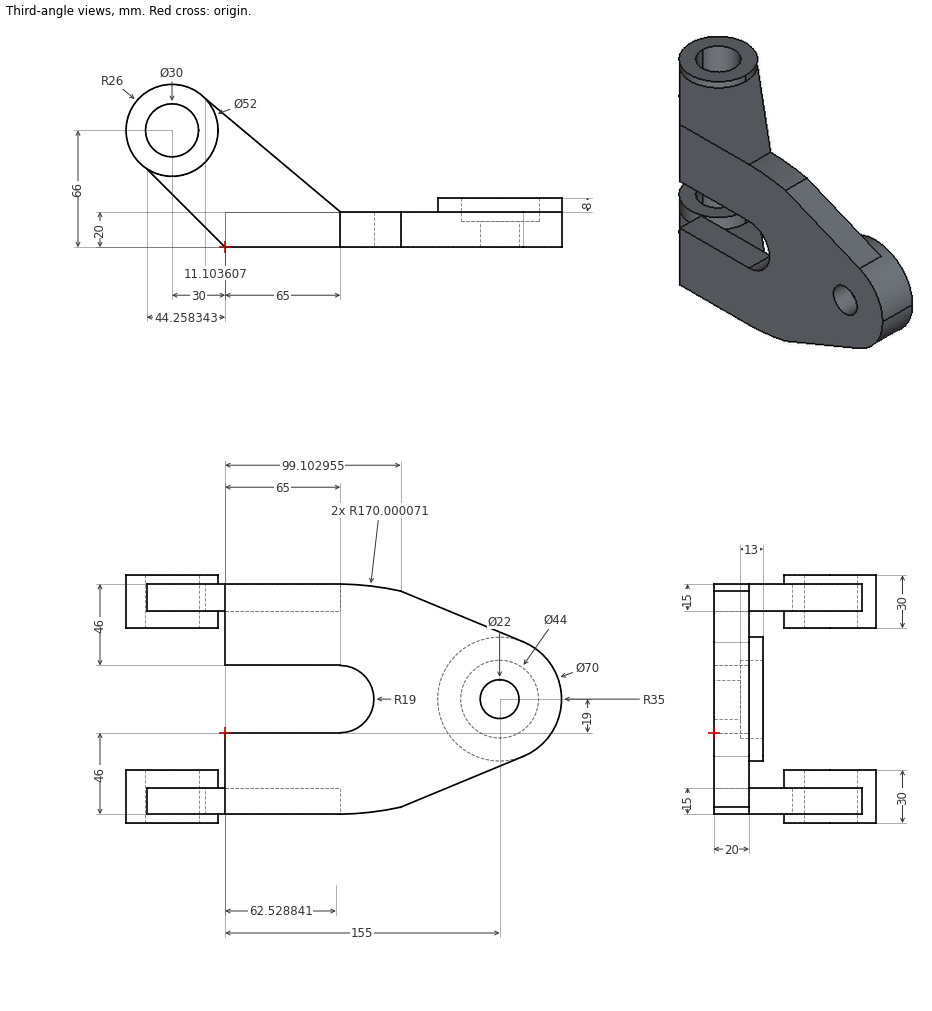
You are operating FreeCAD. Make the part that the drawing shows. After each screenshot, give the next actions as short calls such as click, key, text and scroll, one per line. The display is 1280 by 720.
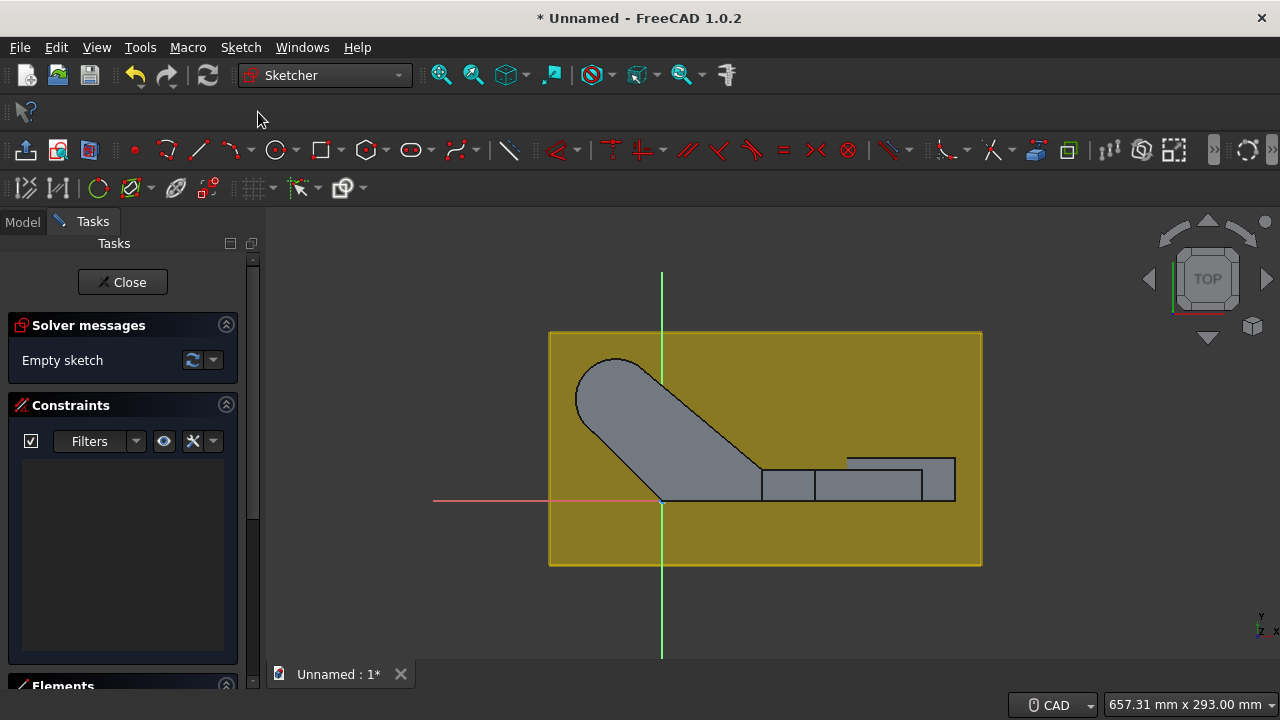
key(q)
key(s)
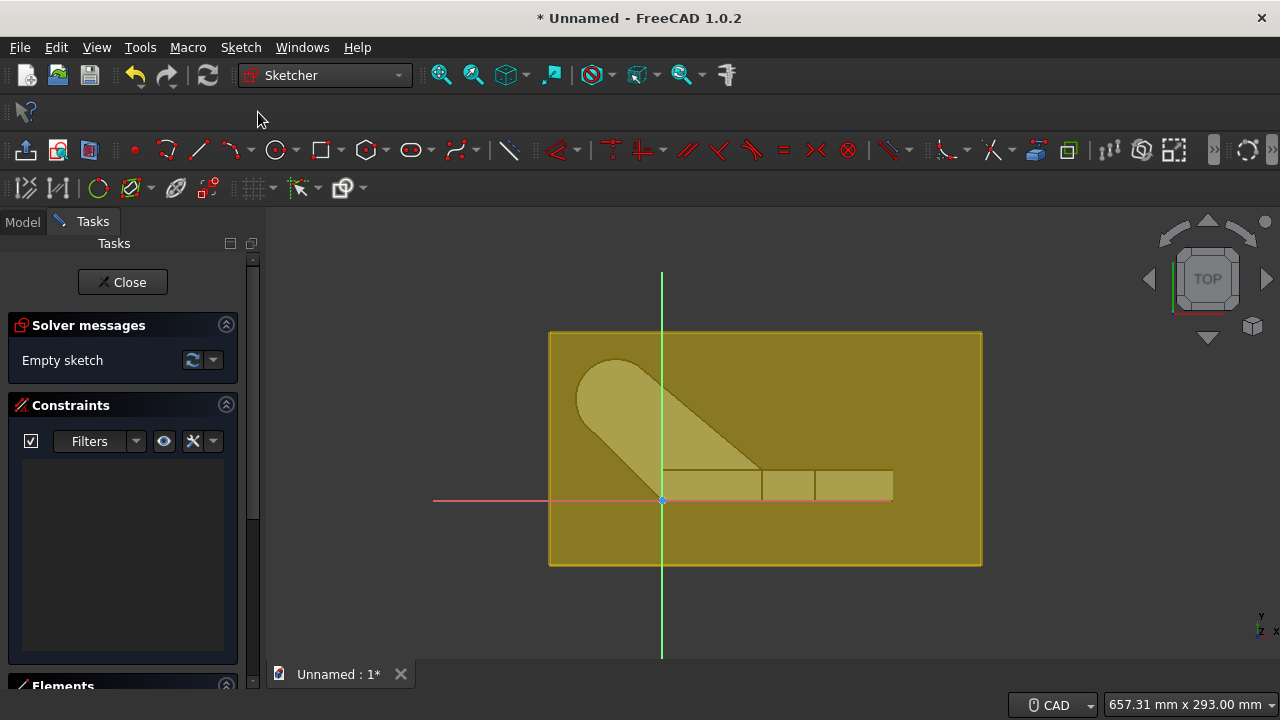
scroll(515, 426, up, 3)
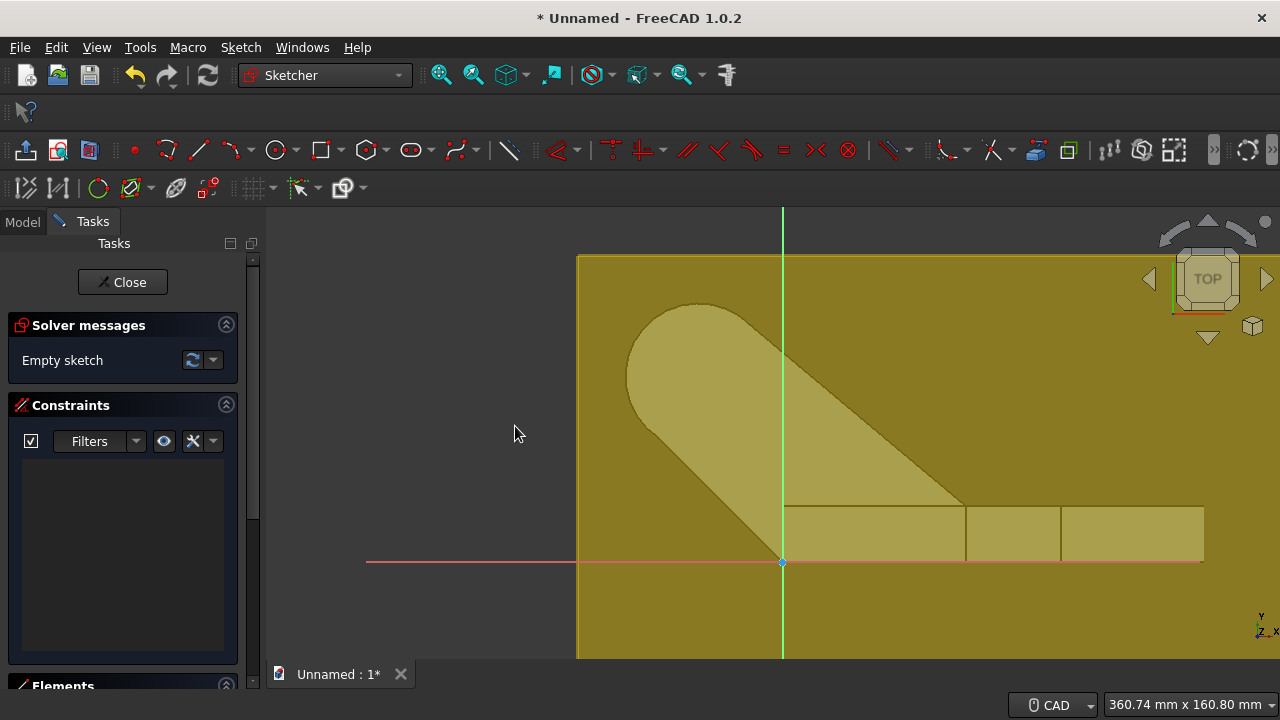
click(276, 150)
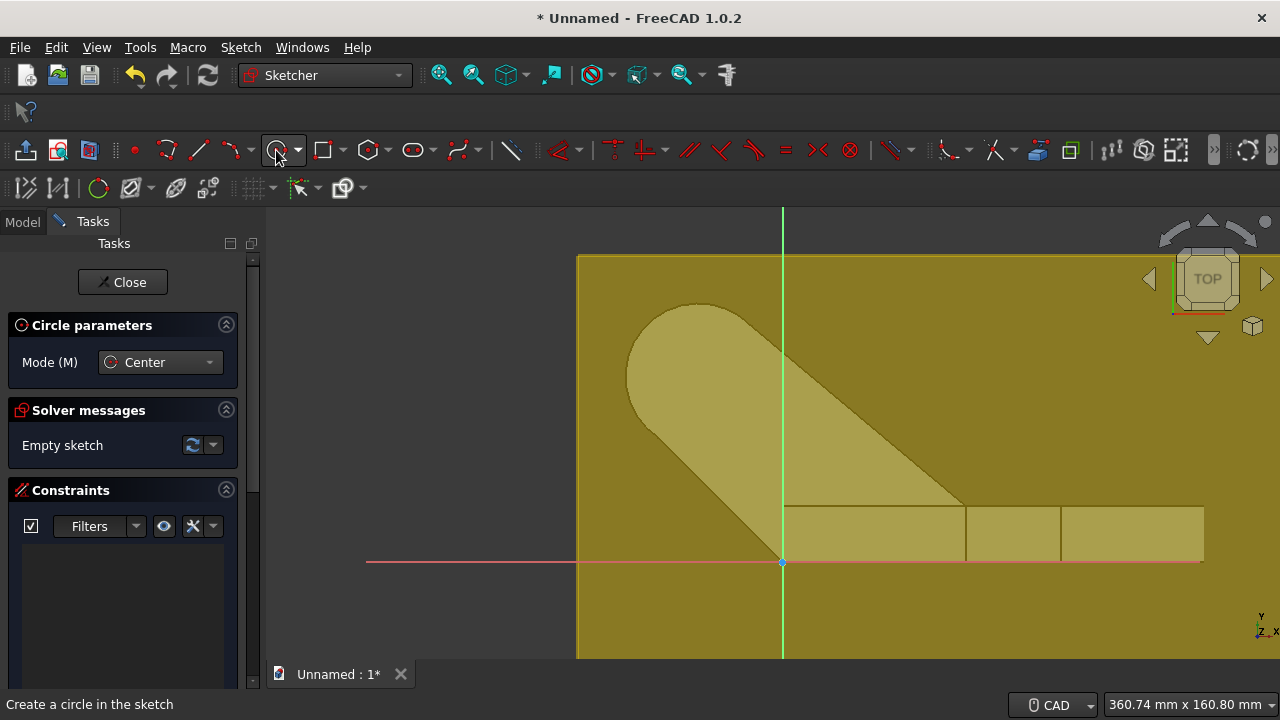
click(699, 377)
move(750, 325)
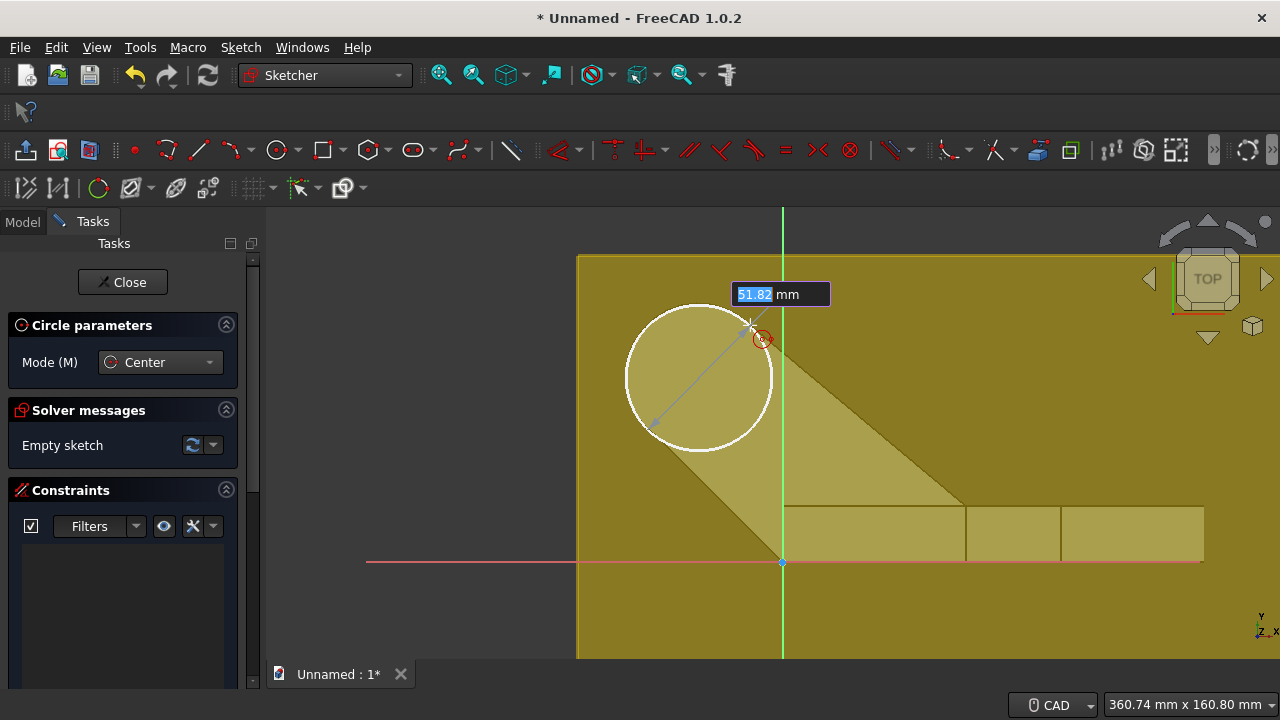
text(52)
key(Return)
key(Escape)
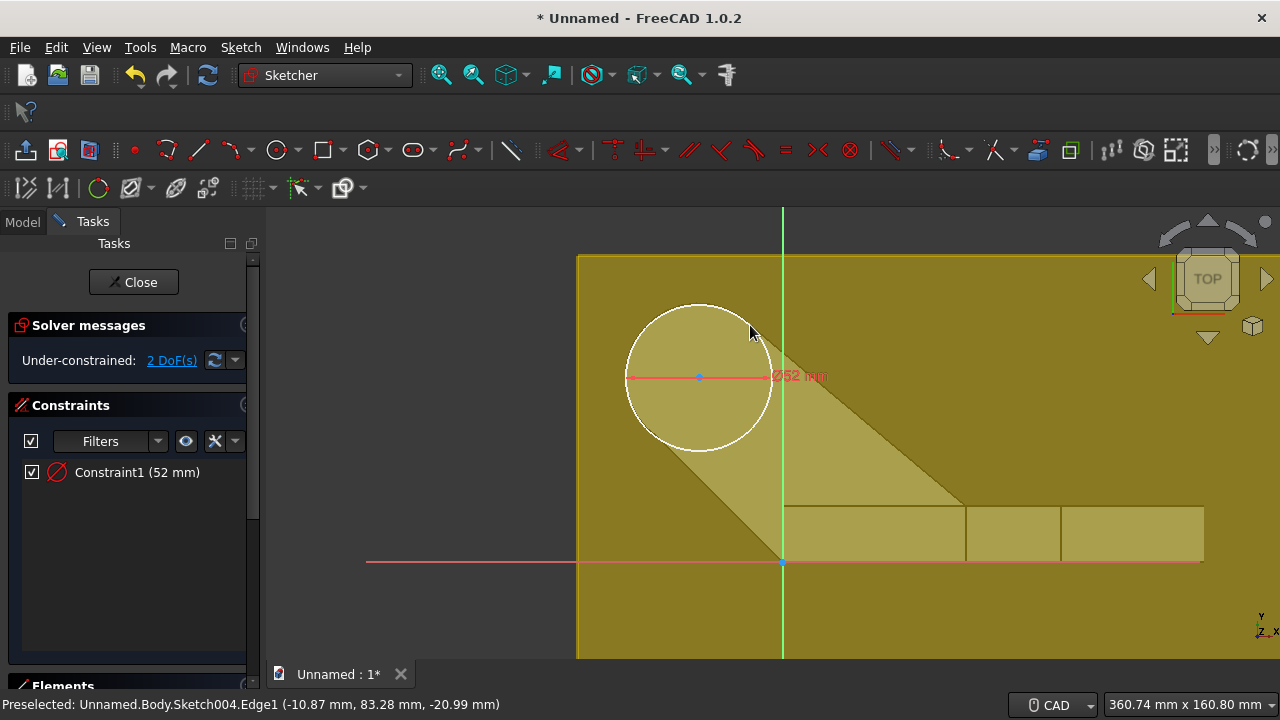
key(d)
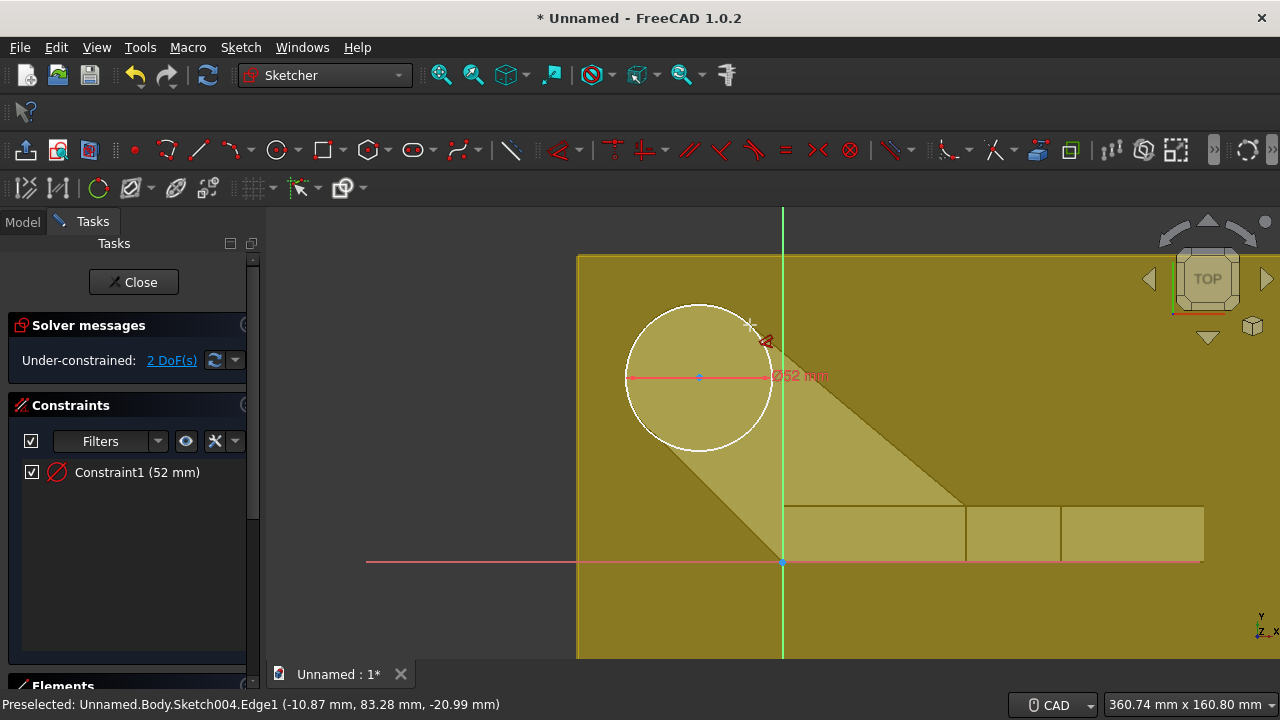
click(699, 378)
click(741, 596)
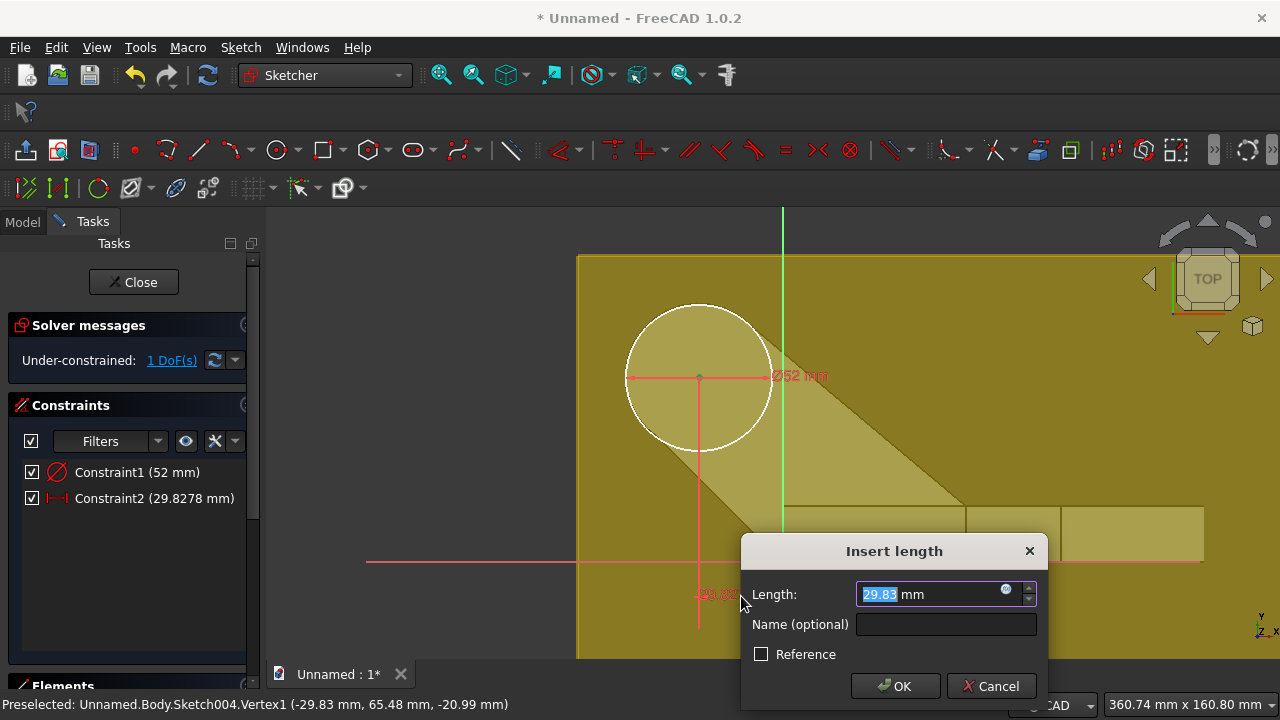
text(30)
key(Return)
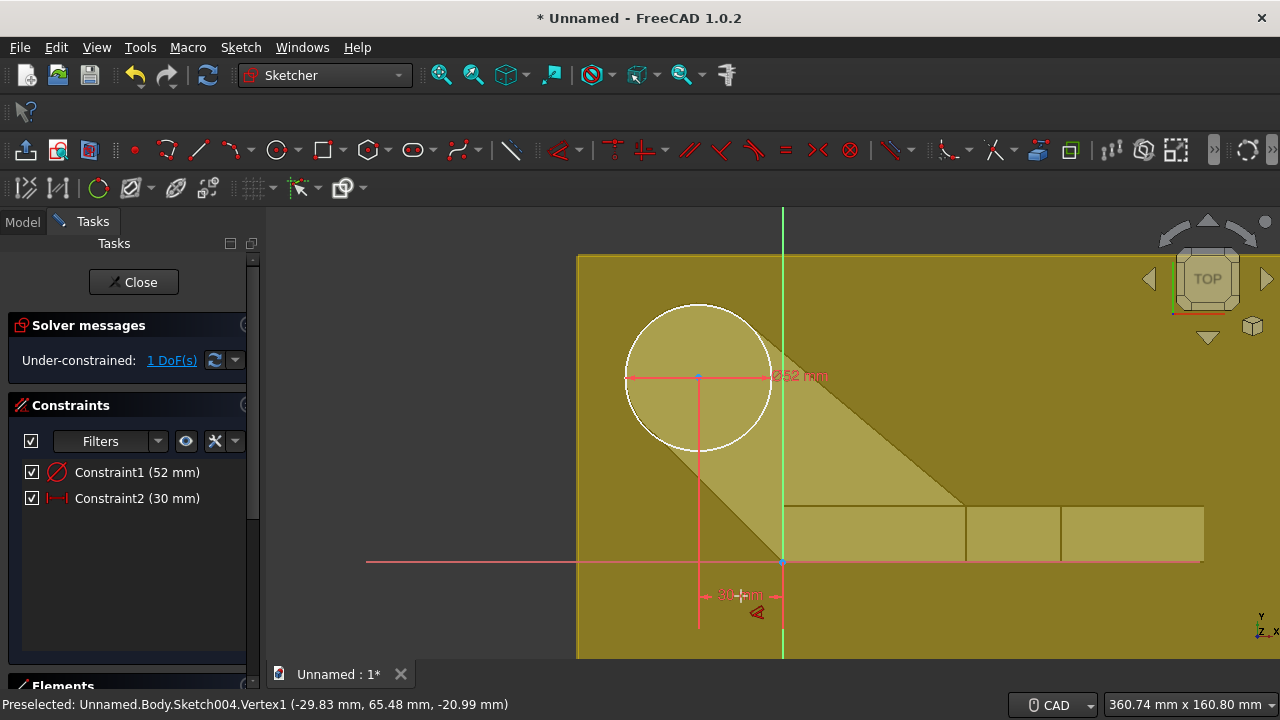
click(699, 378)
click(817, 470)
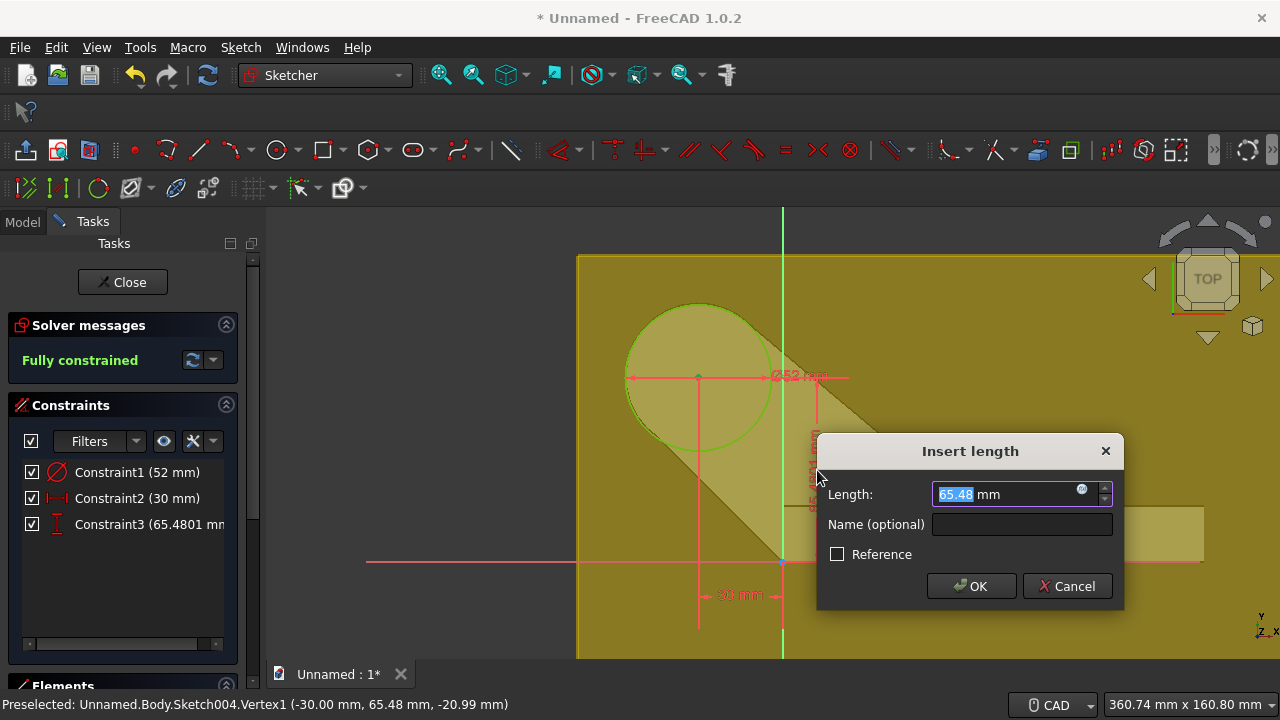
text(66)
key(Return)
key(Escape)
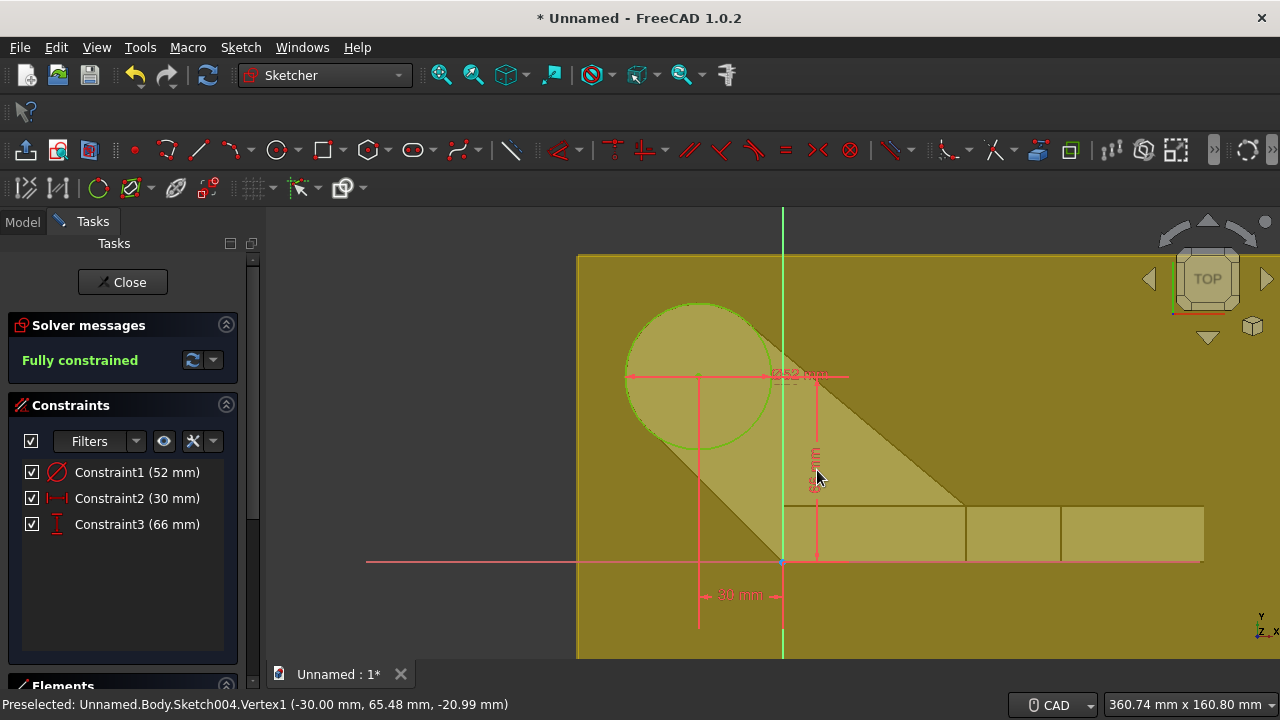
click(123, 282)